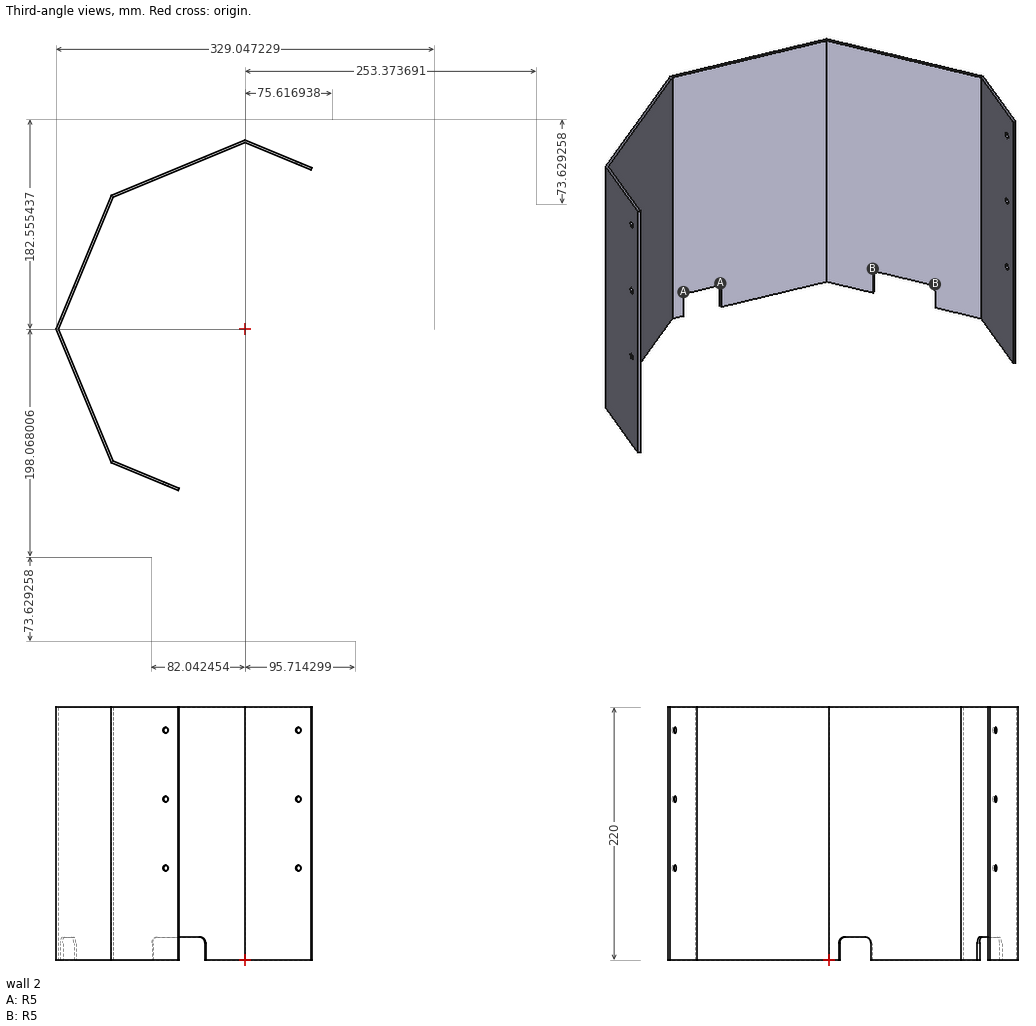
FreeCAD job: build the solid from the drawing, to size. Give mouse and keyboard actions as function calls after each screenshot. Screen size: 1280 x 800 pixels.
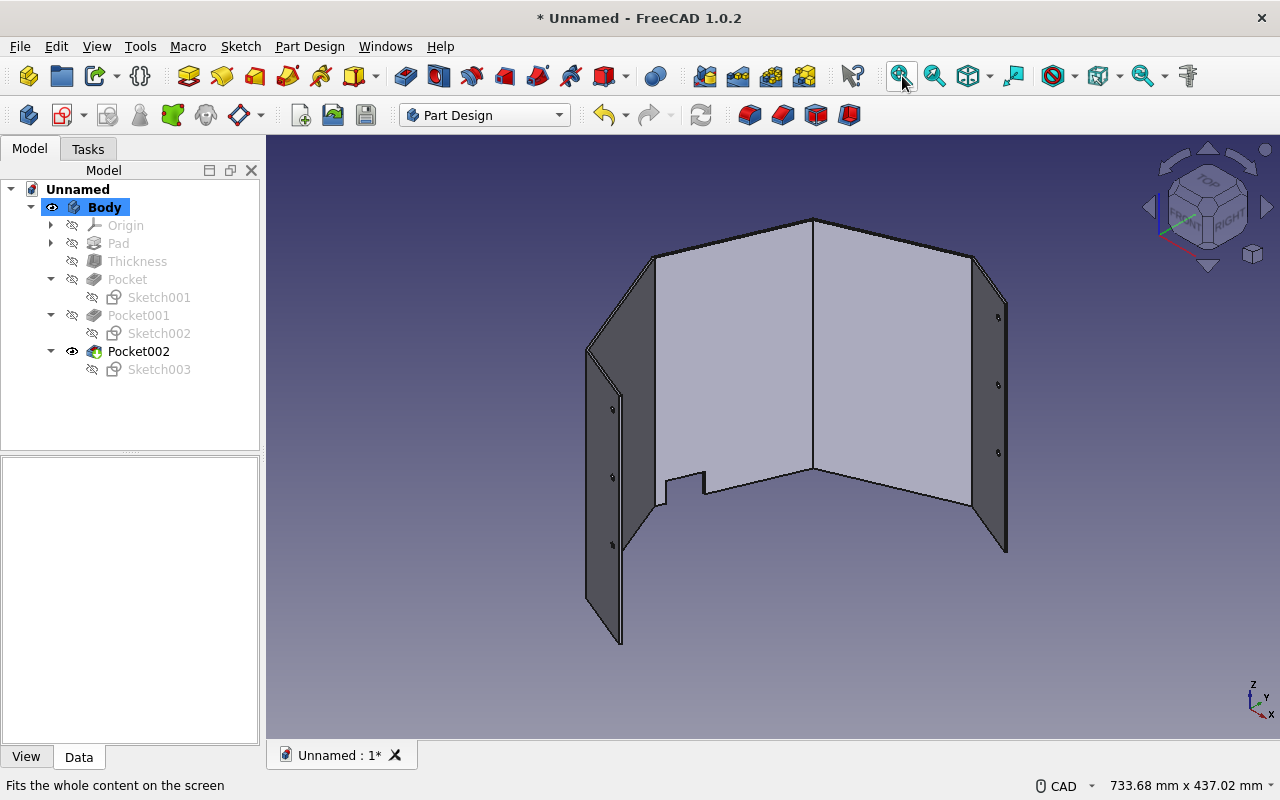
scroll(704, 470, up, 14)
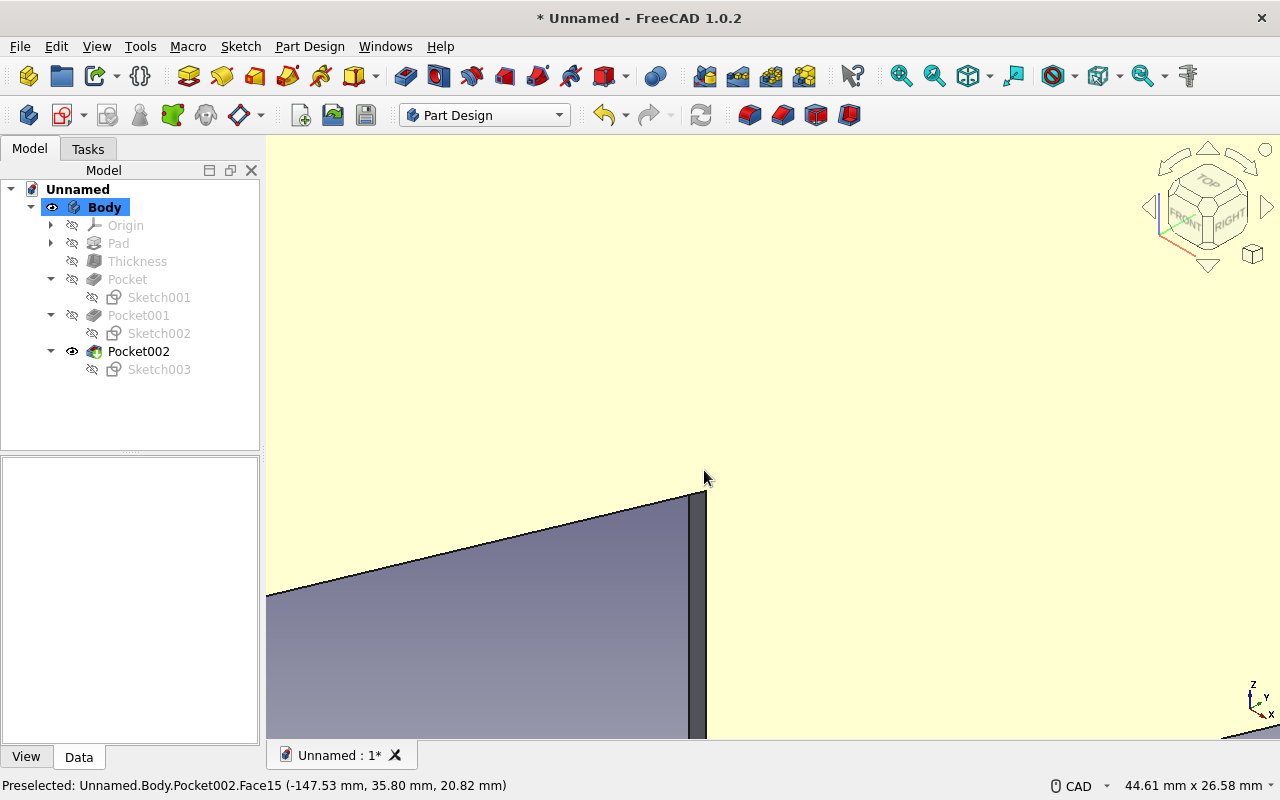
click(902, 76)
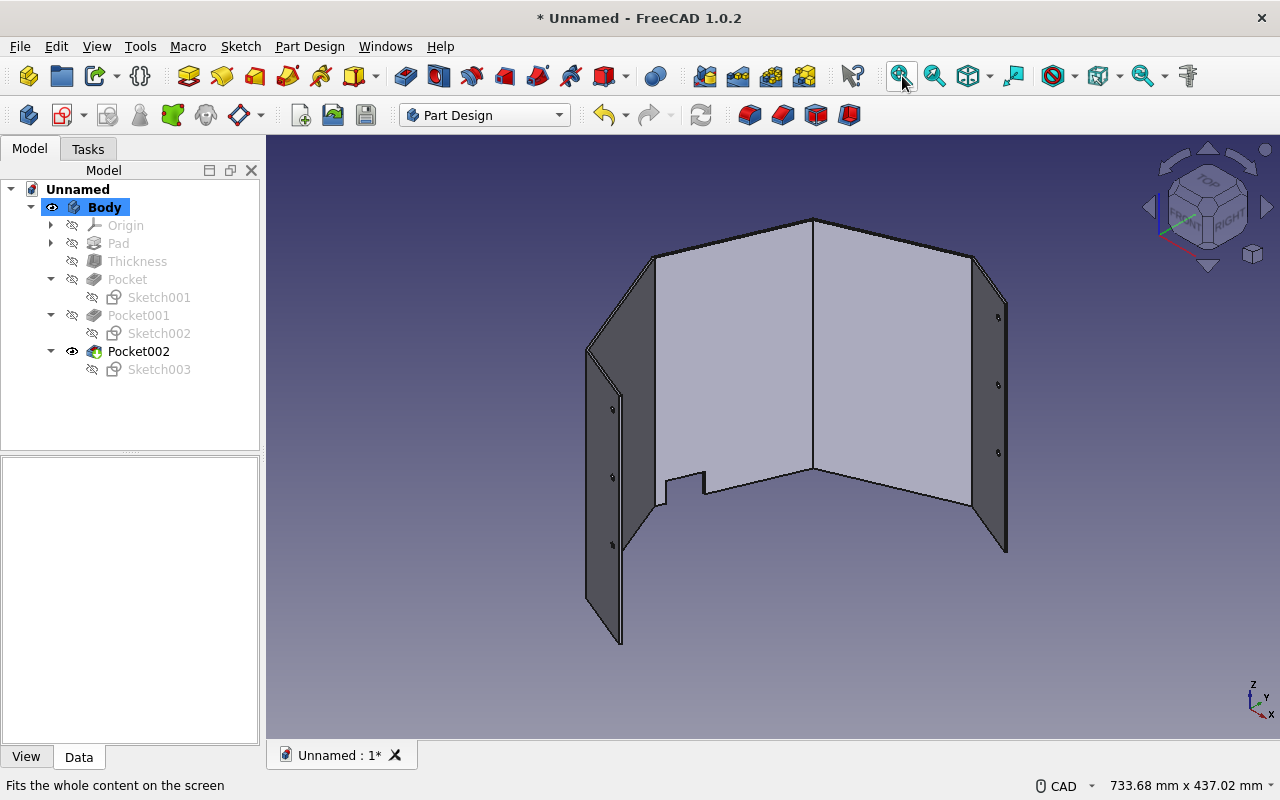
key(2)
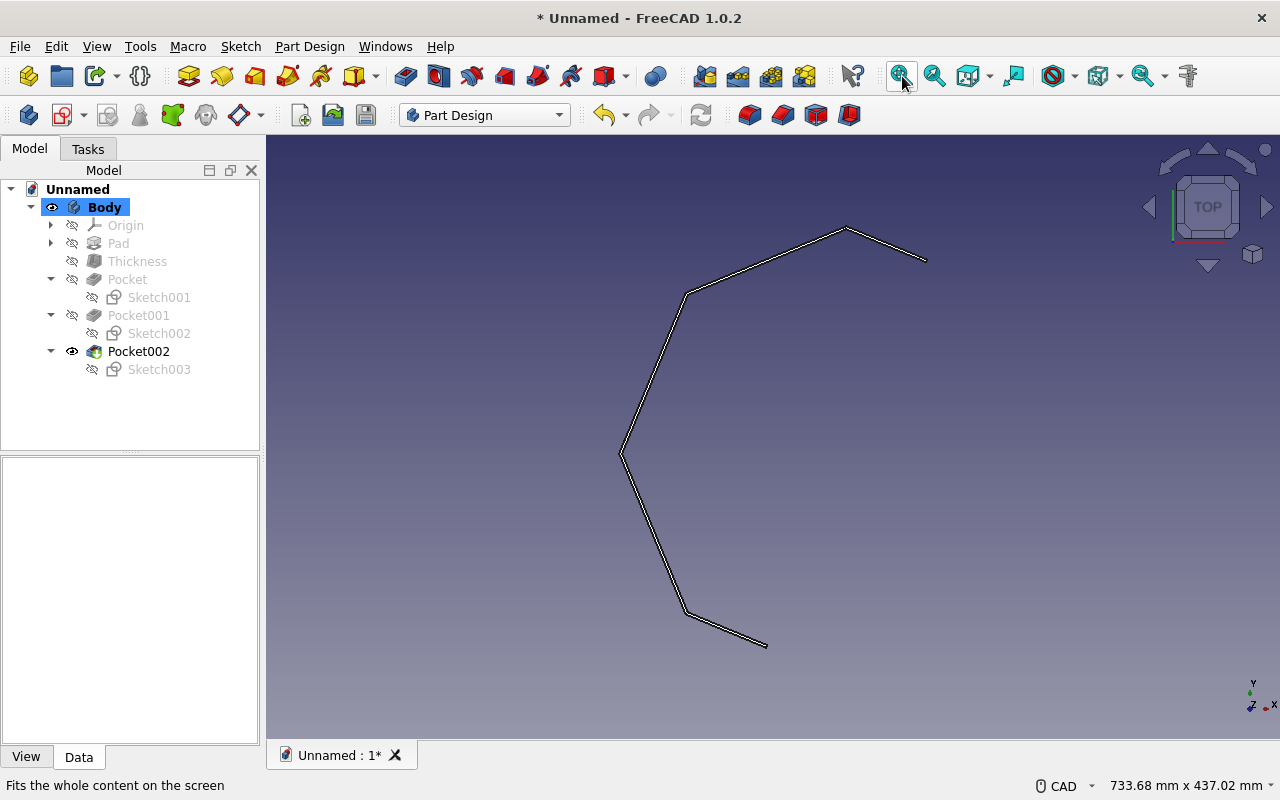
scroll(642, 402, up, 14)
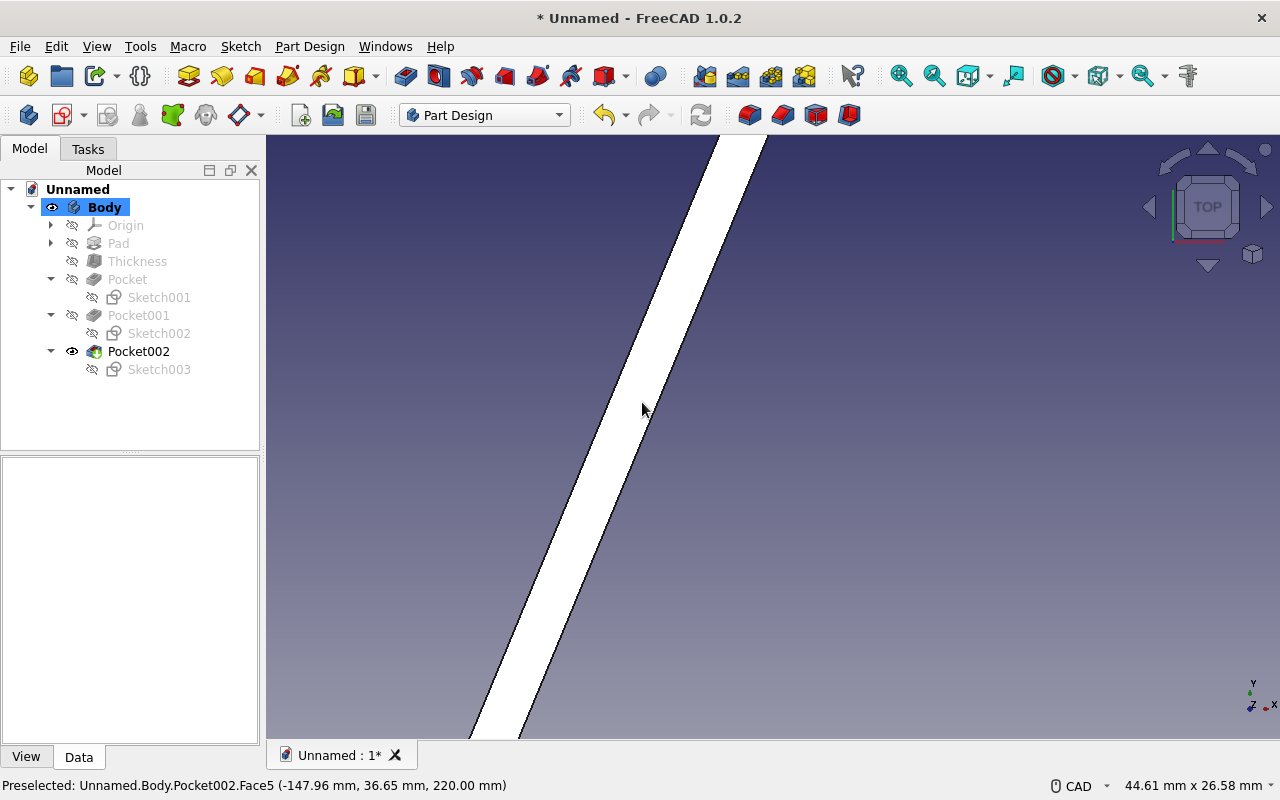
click(902, 76)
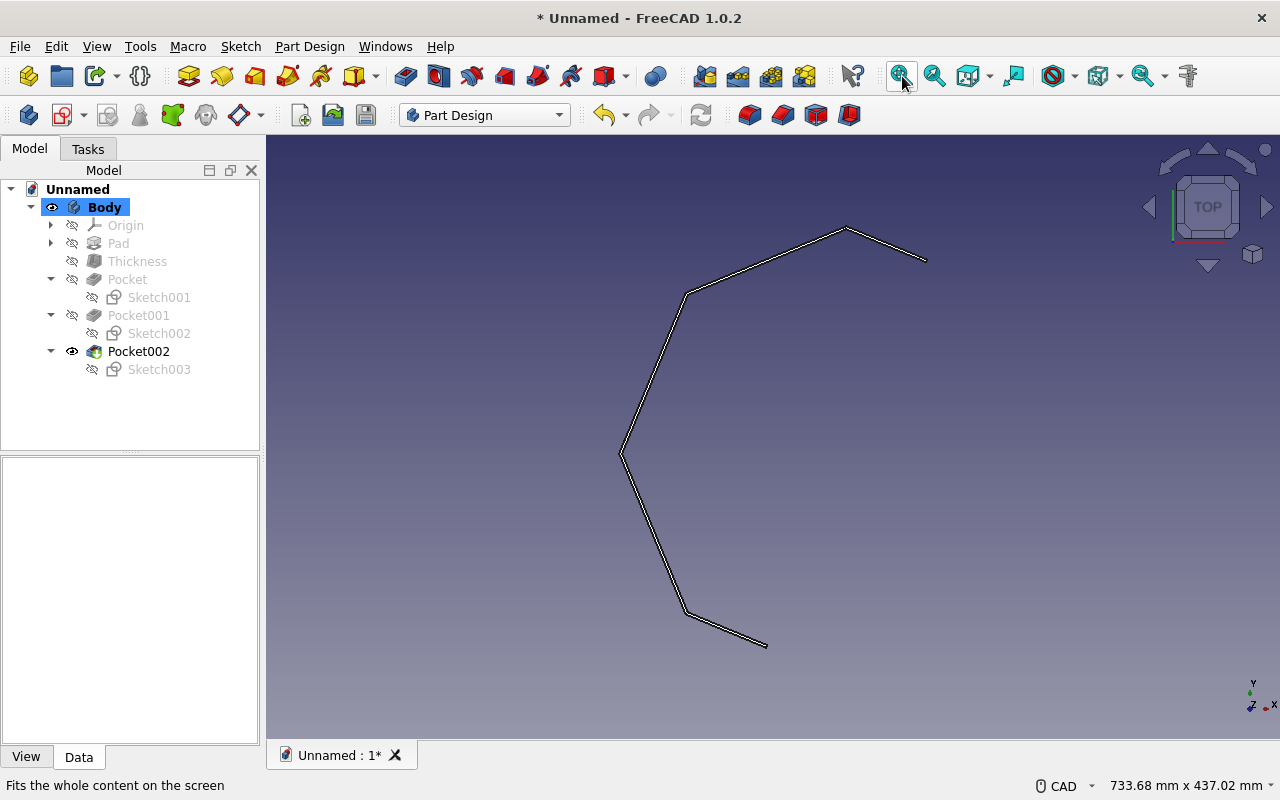
key(1)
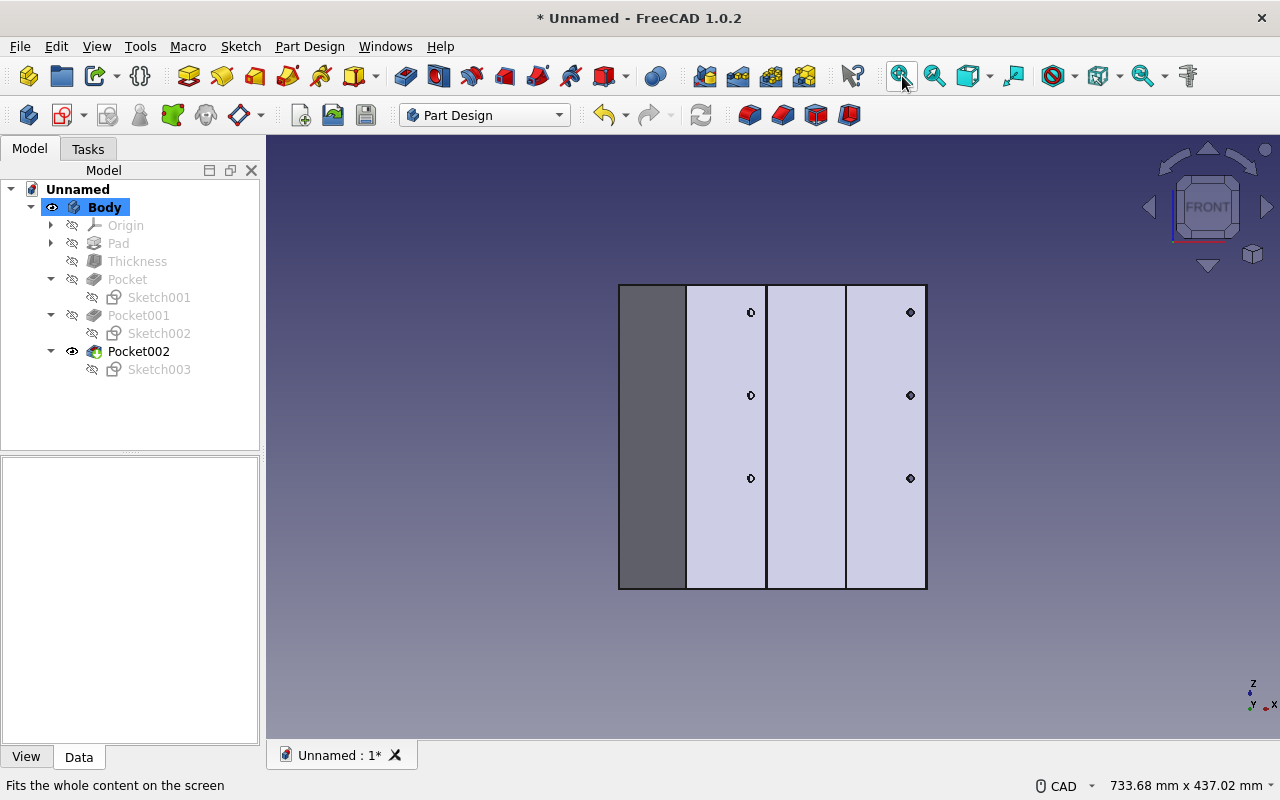
scroll(642, 560, up, 14)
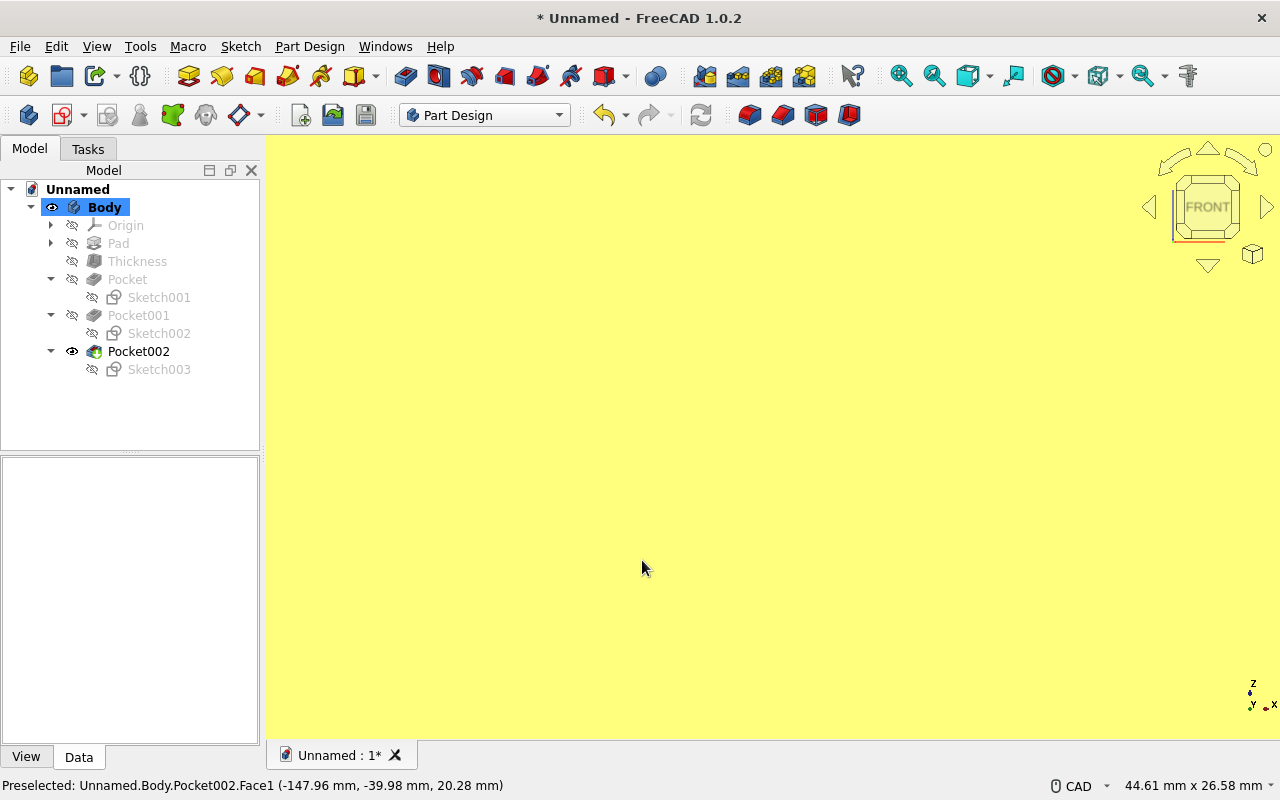
click(902, 76)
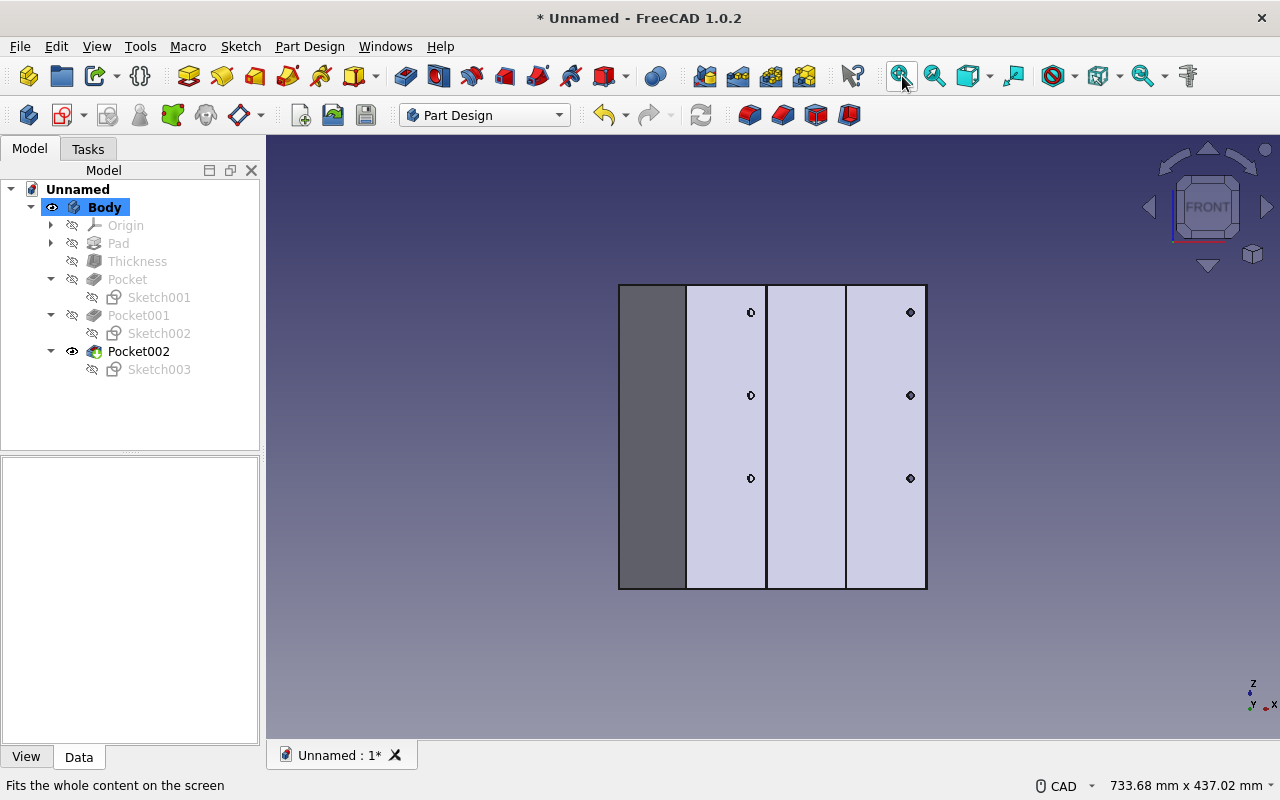
key(3)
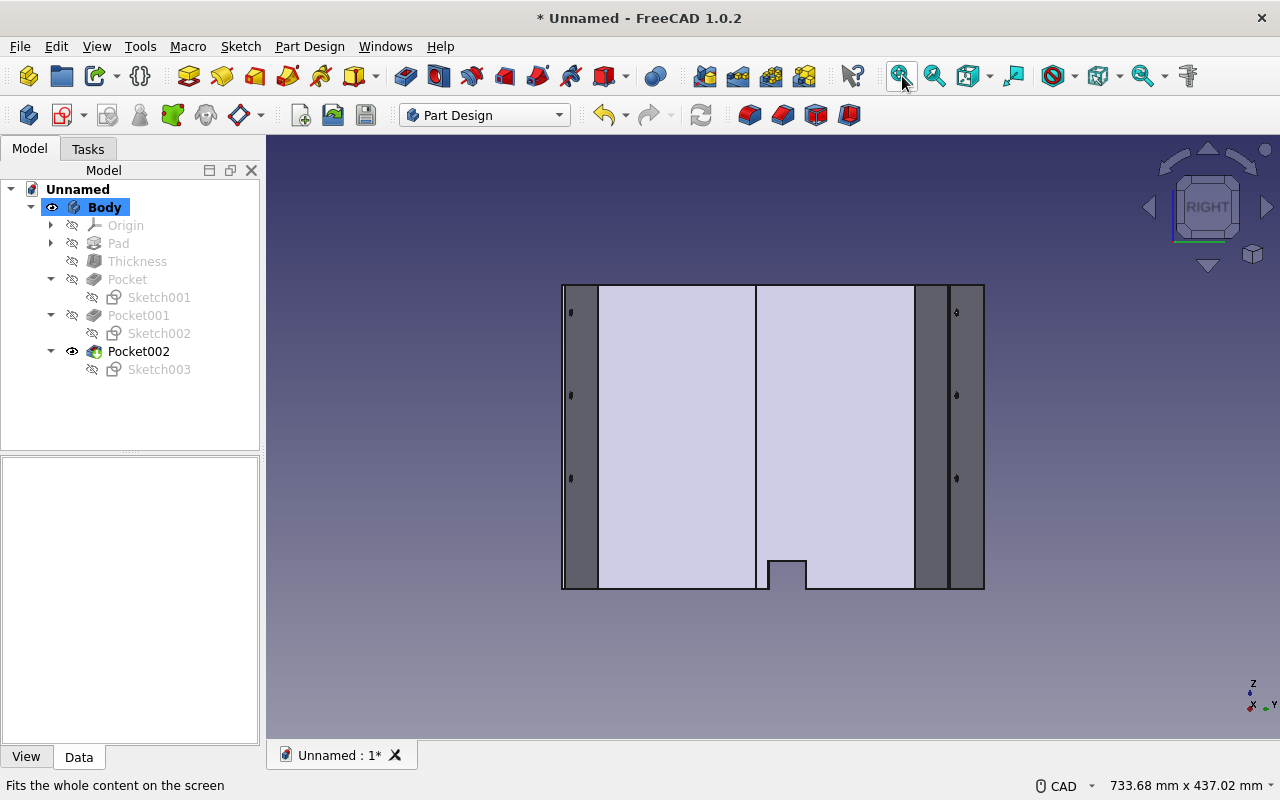
scroll(807, 560, up, 14)